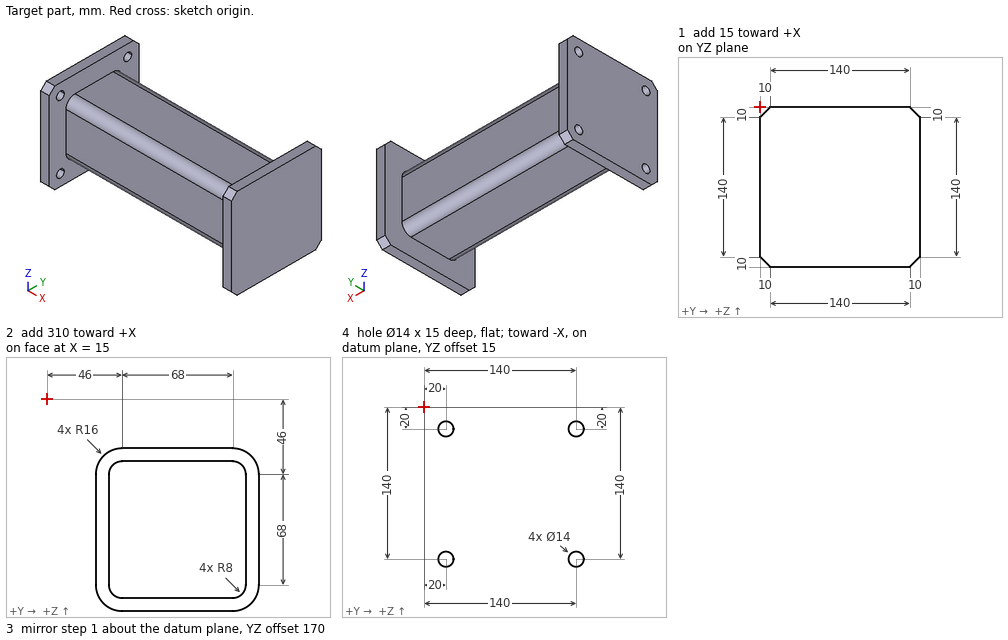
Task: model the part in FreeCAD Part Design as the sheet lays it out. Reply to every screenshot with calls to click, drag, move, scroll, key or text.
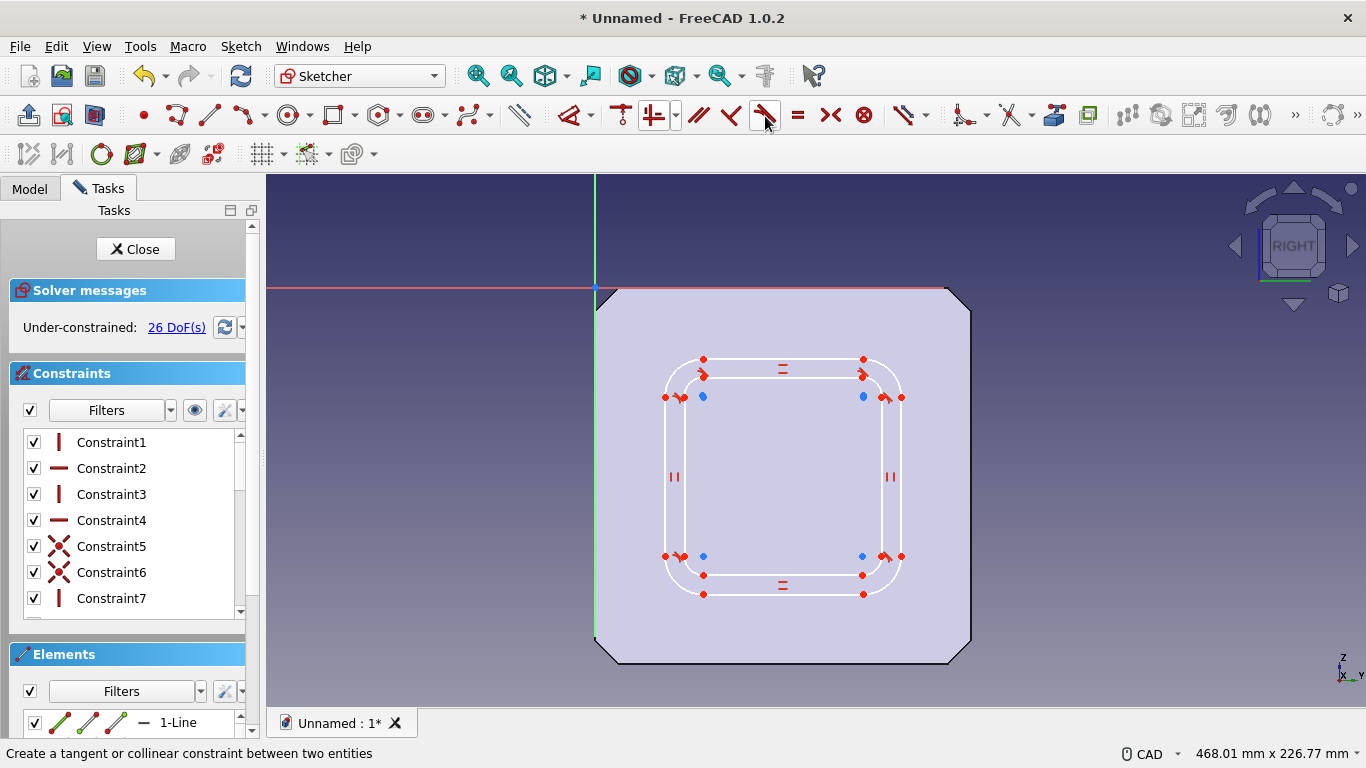
click(751, 595)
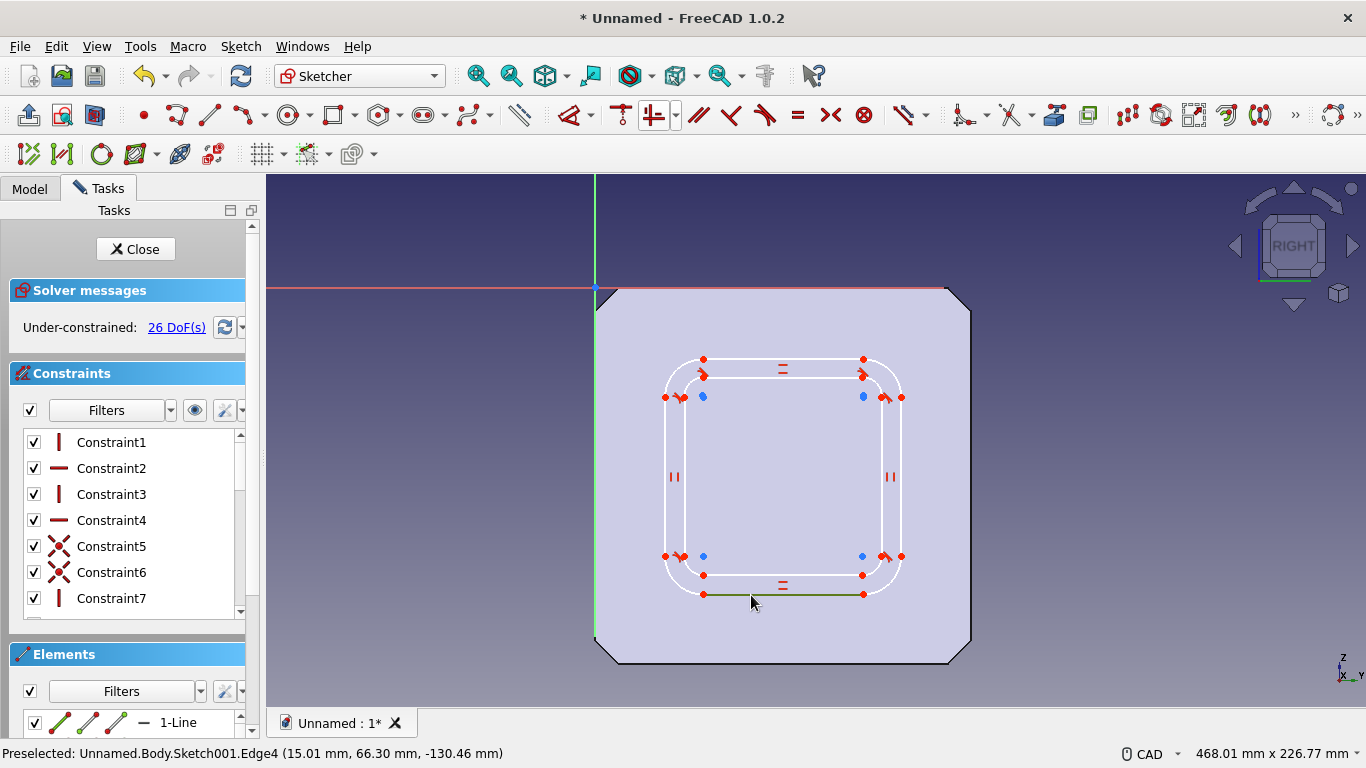
click(669, 573)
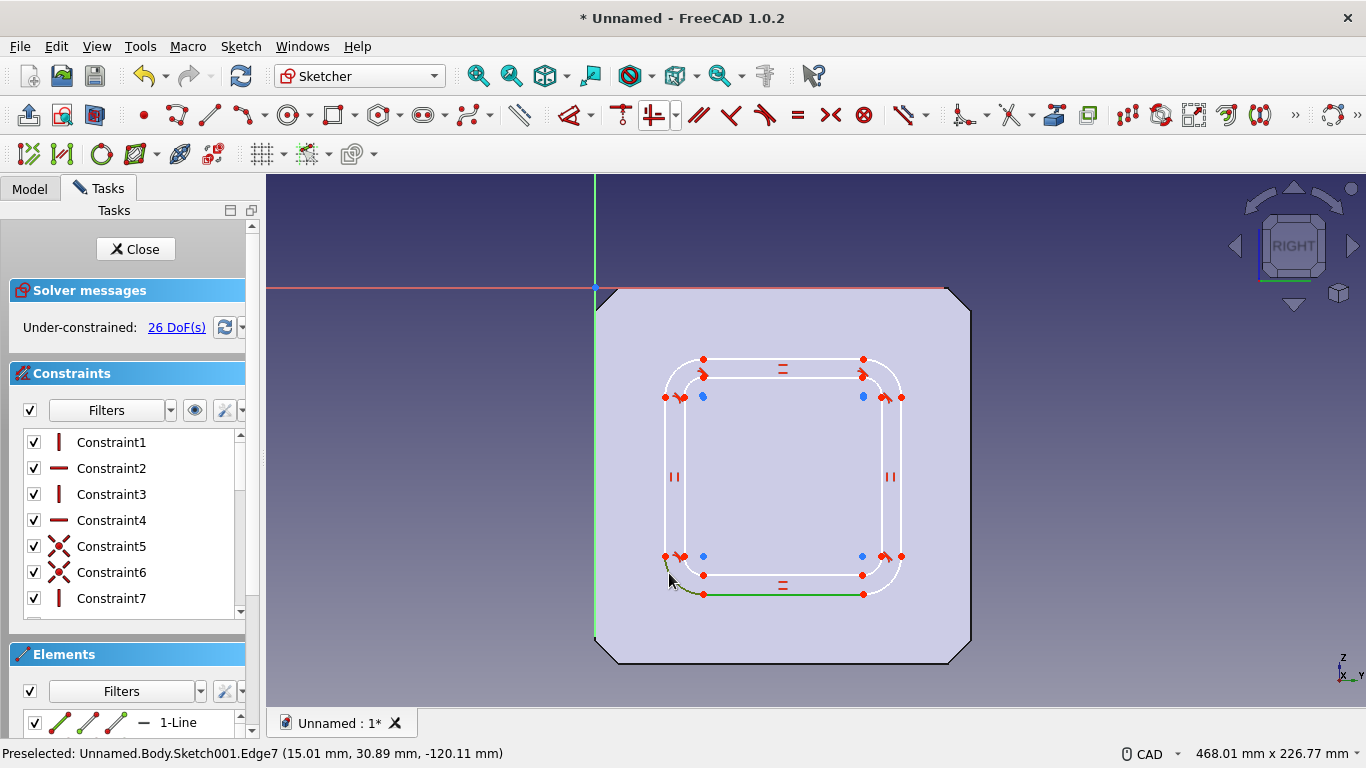
key(t)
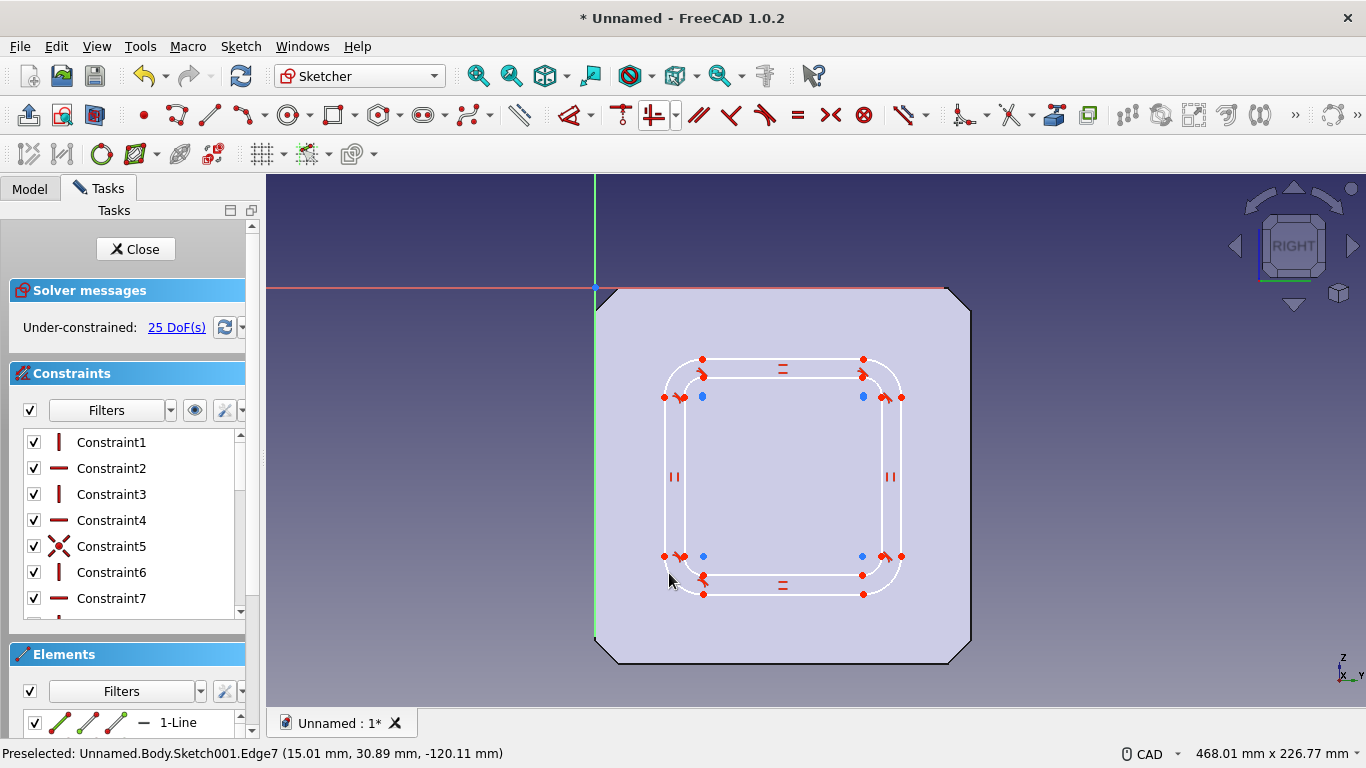
click(751, 595)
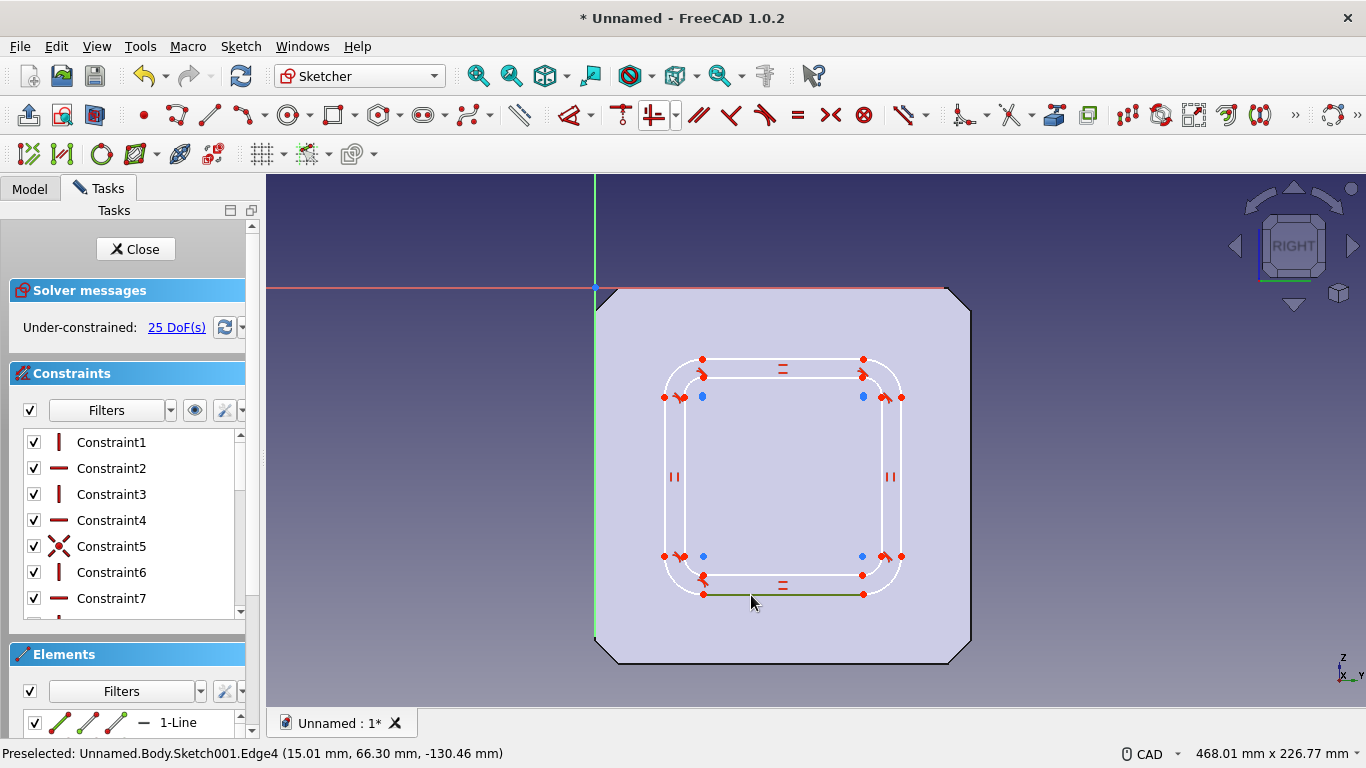
click(880, 590)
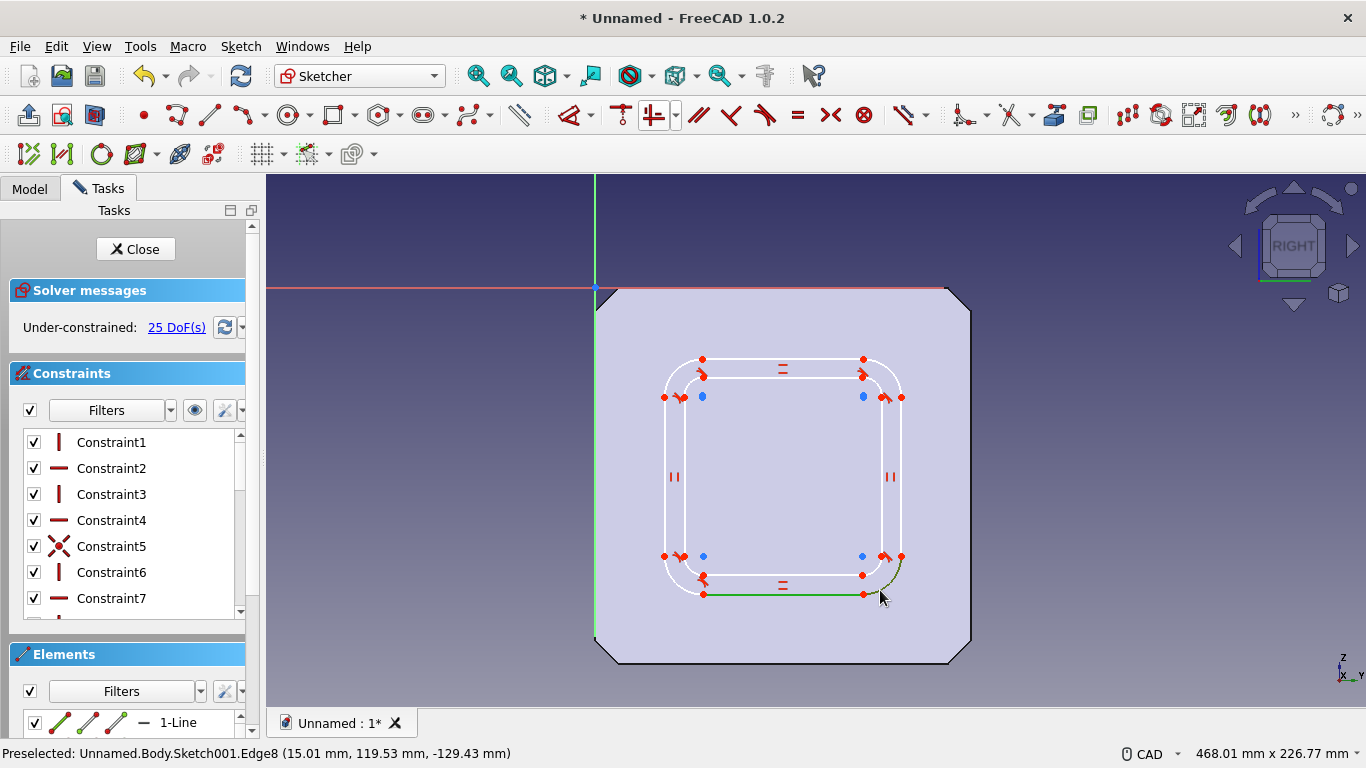
click(765, 116)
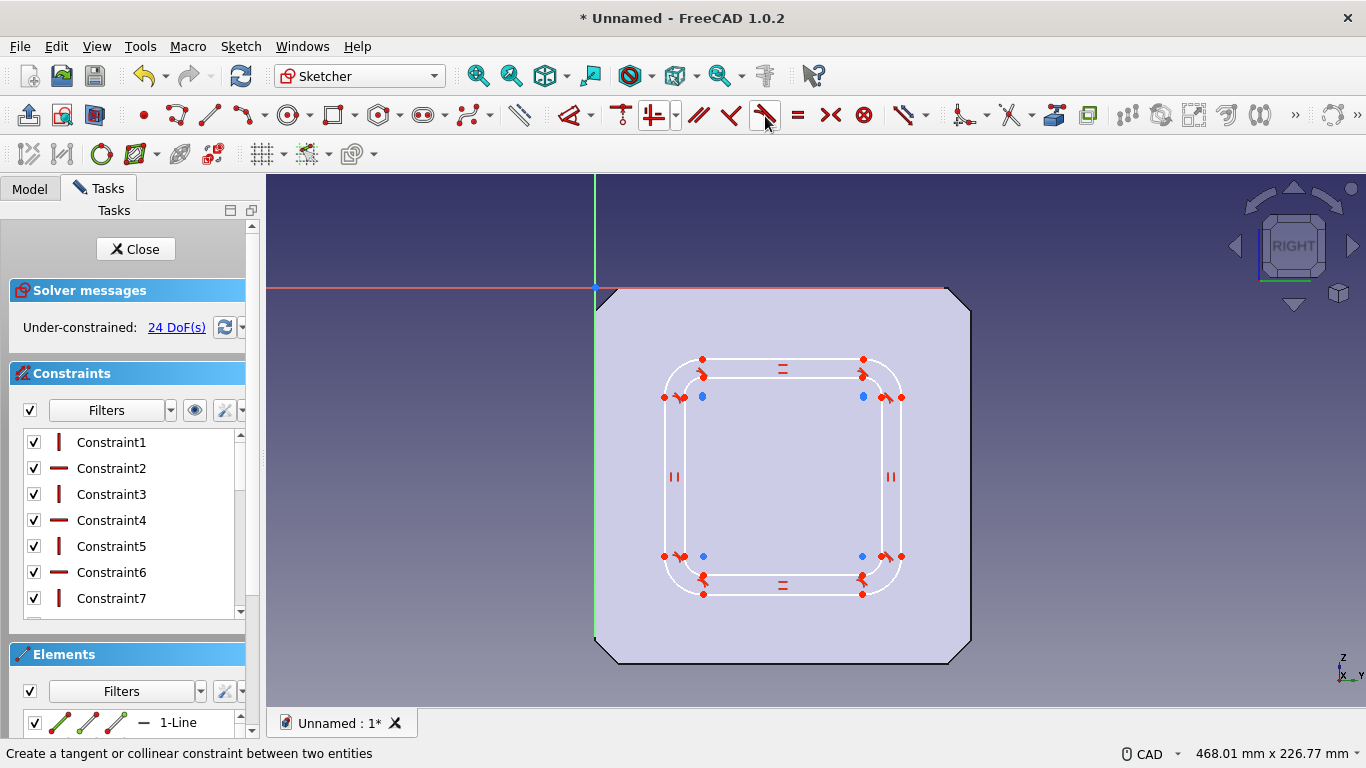
click(882, 445)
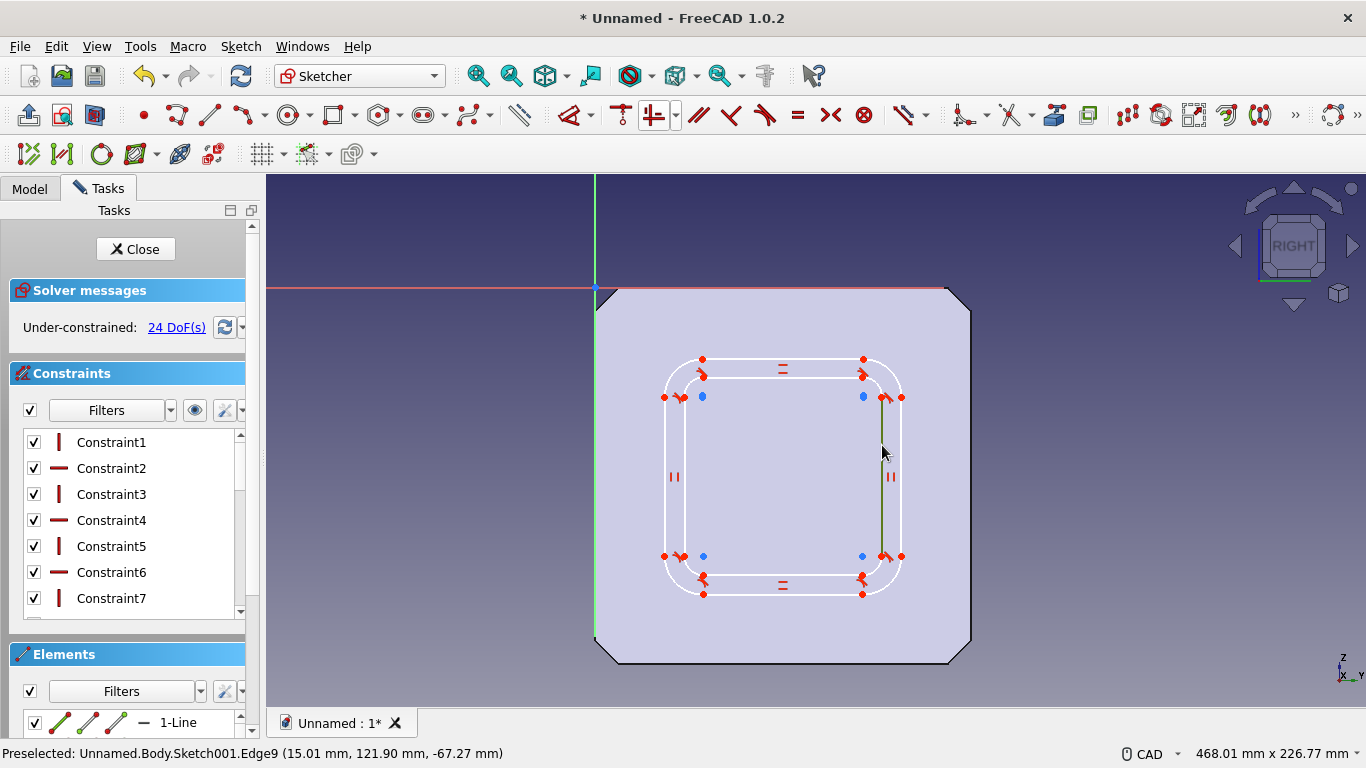
click(876, 570)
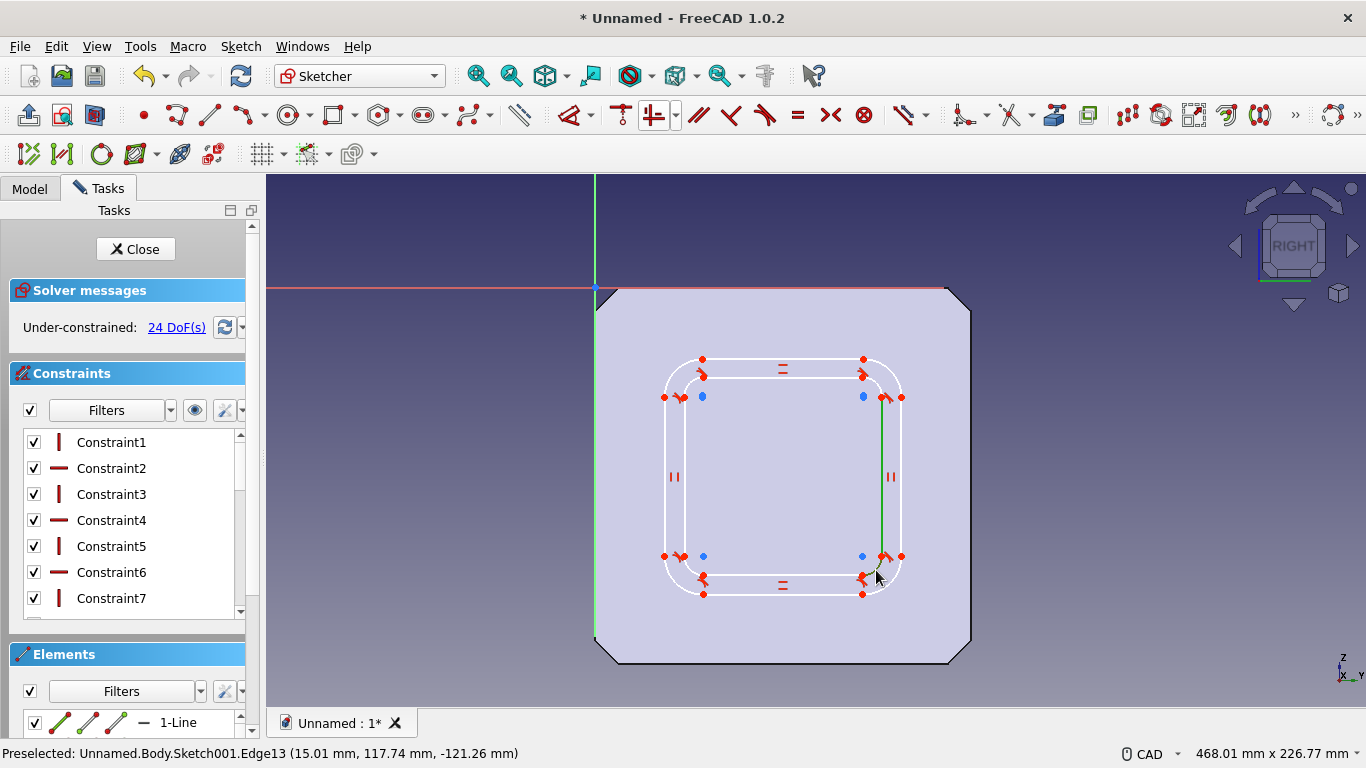
click(765, 116)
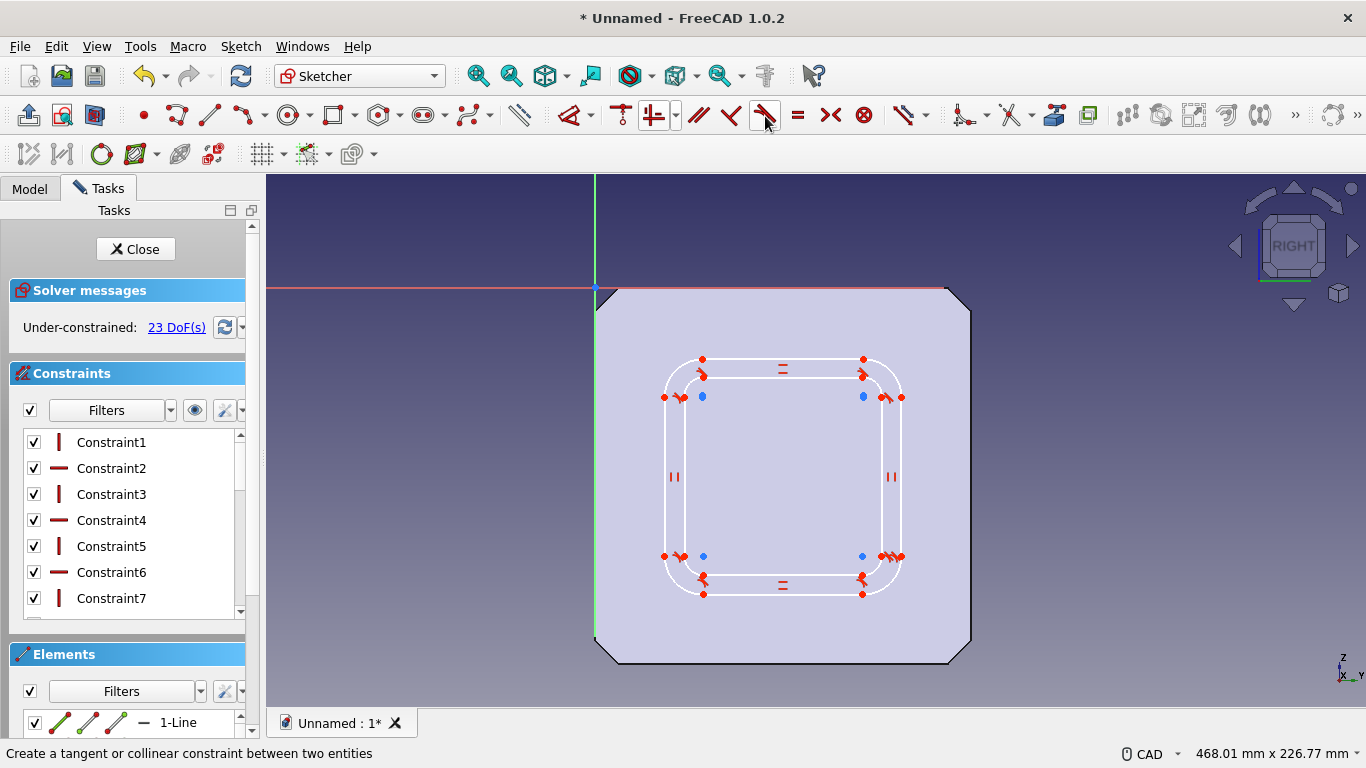
click(882, 445)